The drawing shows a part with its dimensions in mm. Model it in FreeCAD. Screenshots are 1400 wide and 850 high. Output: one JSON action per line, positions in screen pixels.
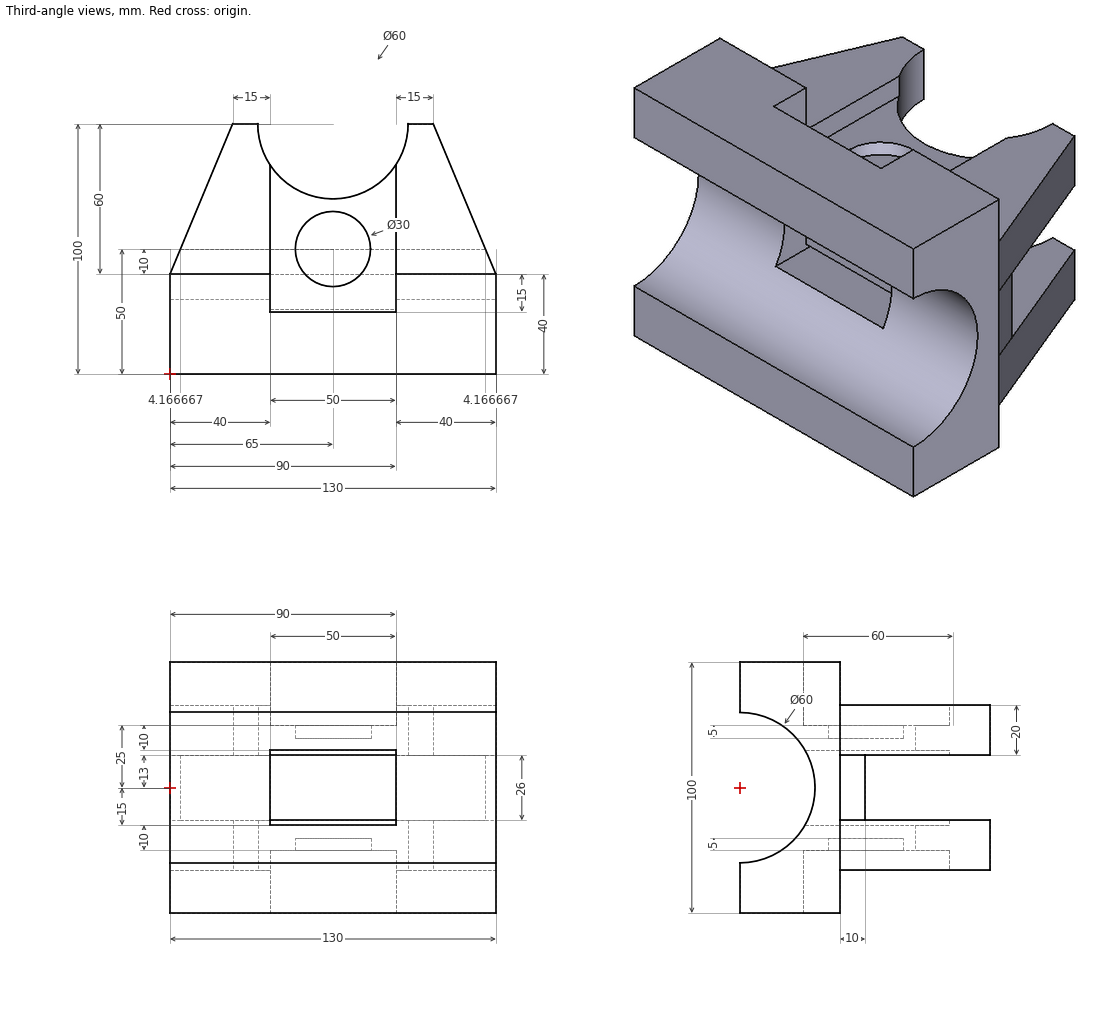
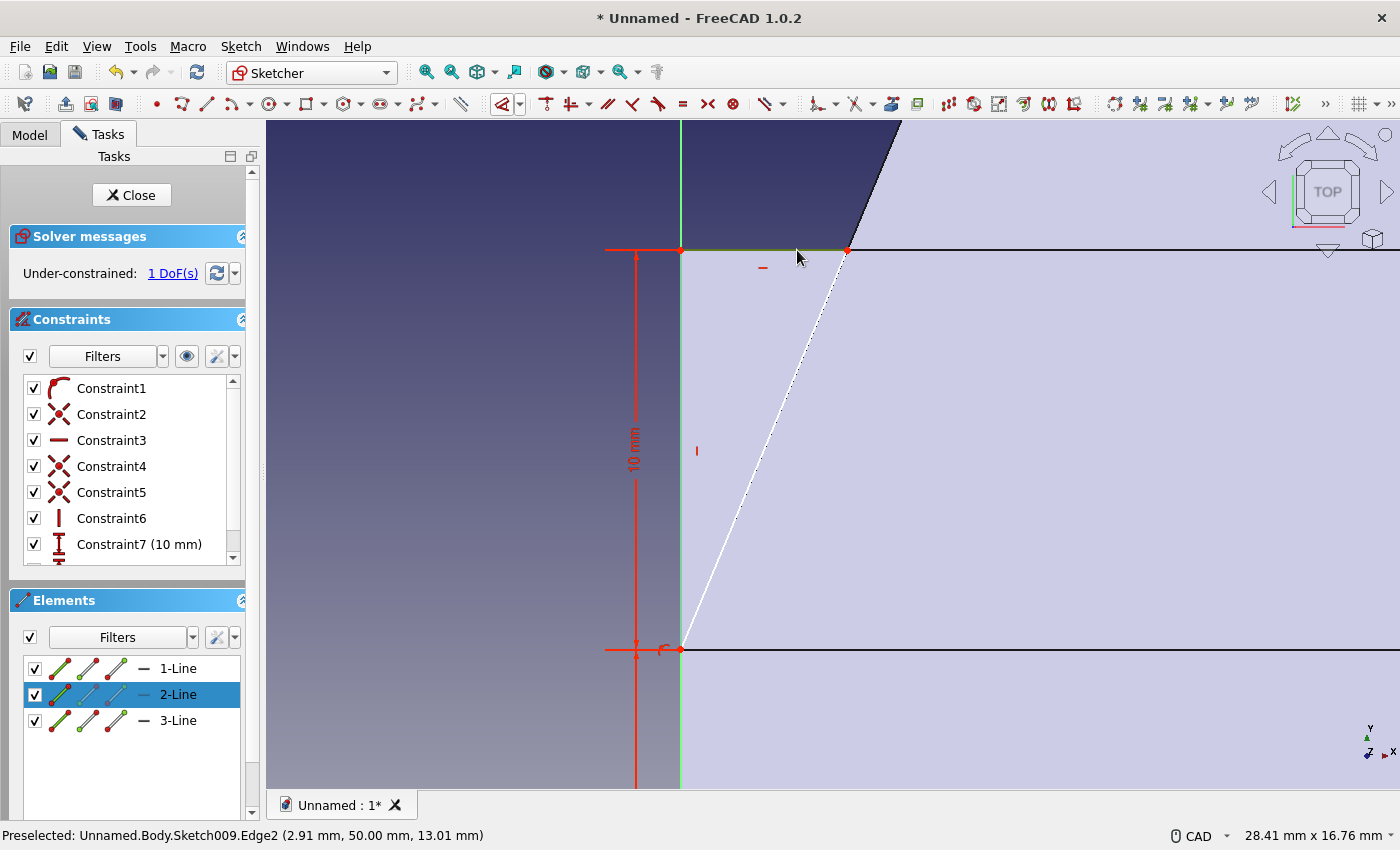
{"action": "left_click", "coordinate": [520, 104]}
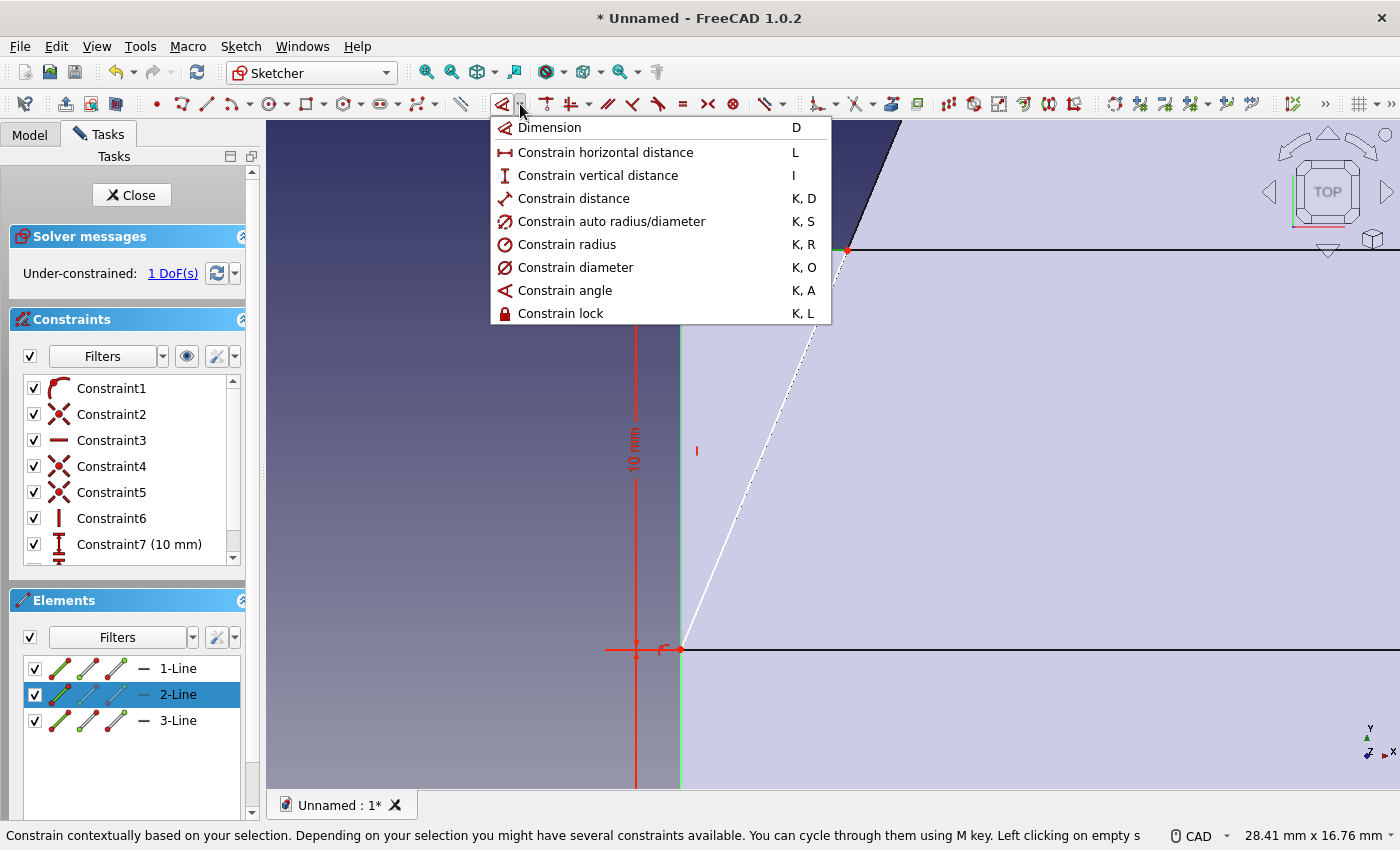
{"action": "left_click", "coordinate": [661, 152]}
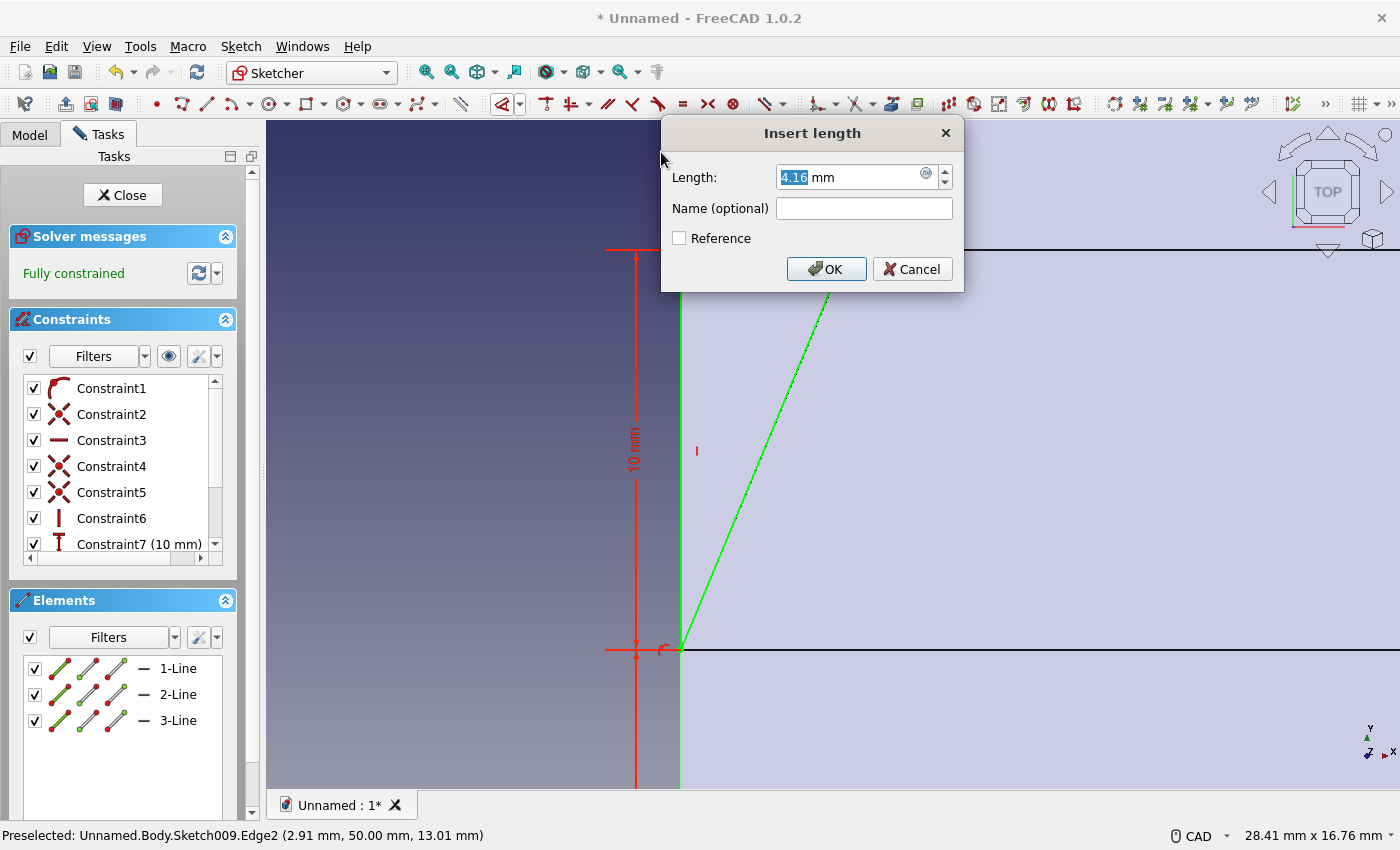
{"action": "type", "text": "4.166667"}
{"action": "key", "text": "Return"}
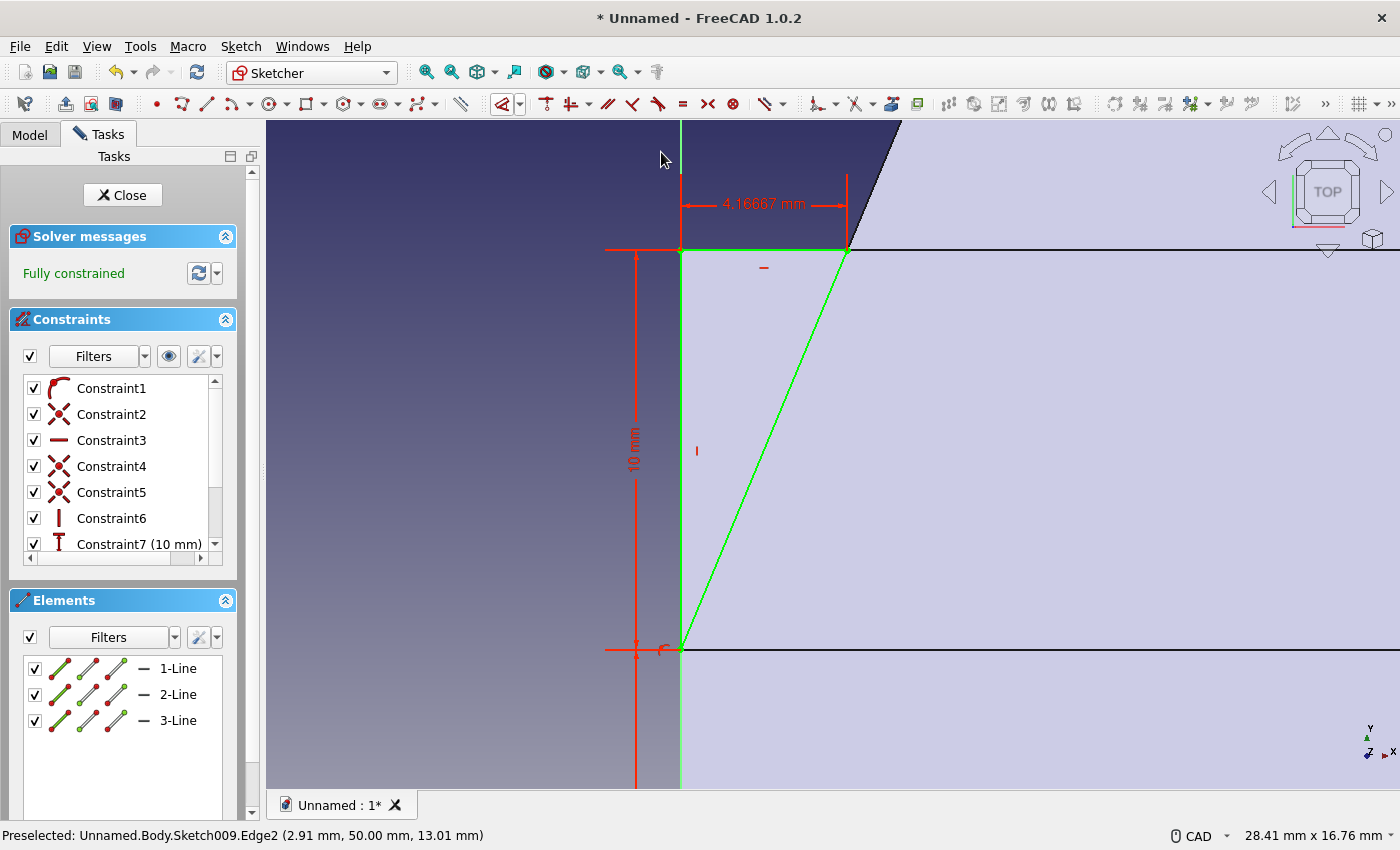
{"action": "left_click", "coordinate": [123, 195]}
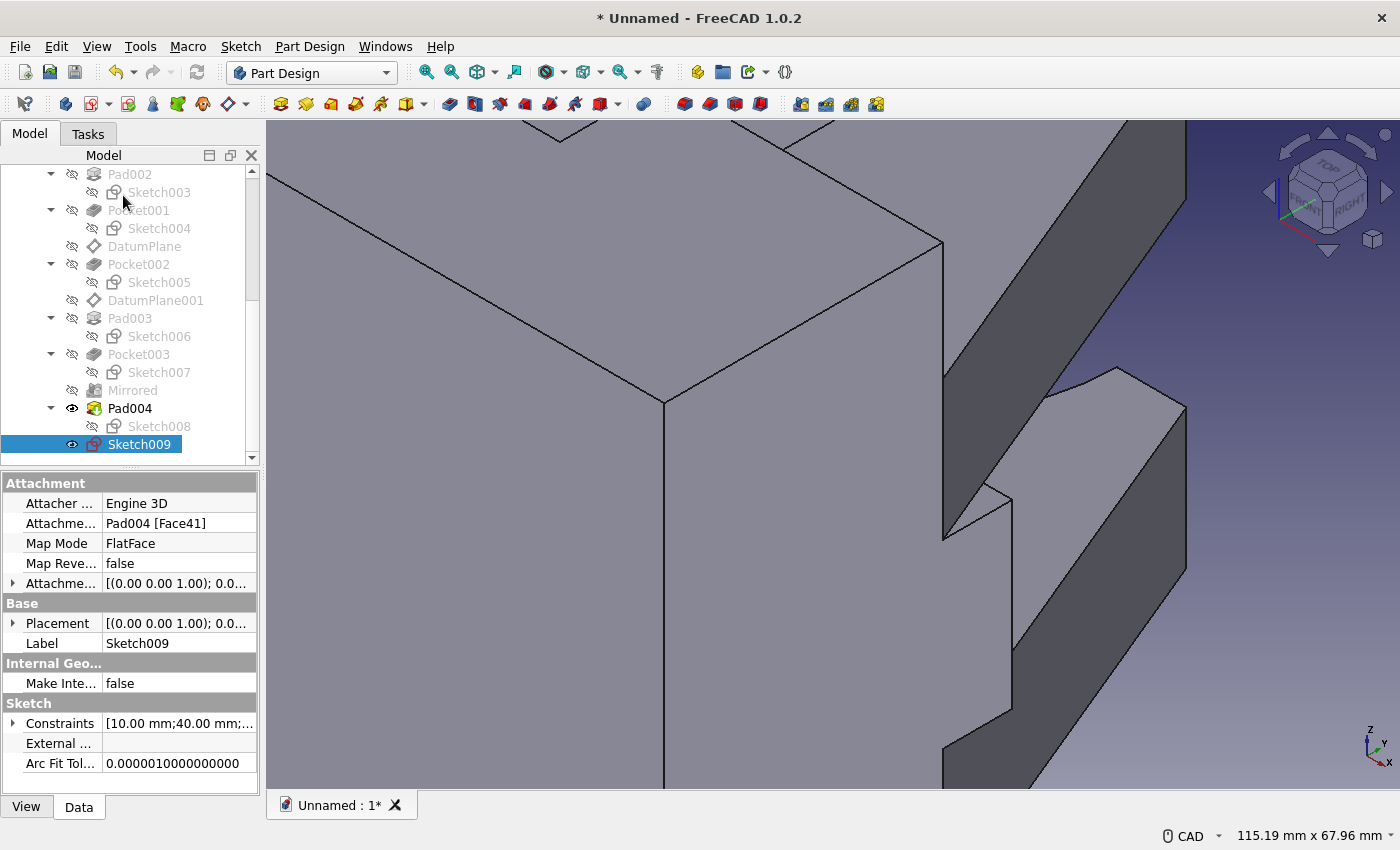
{"action": "left_click", "coordinate": [450, 104]}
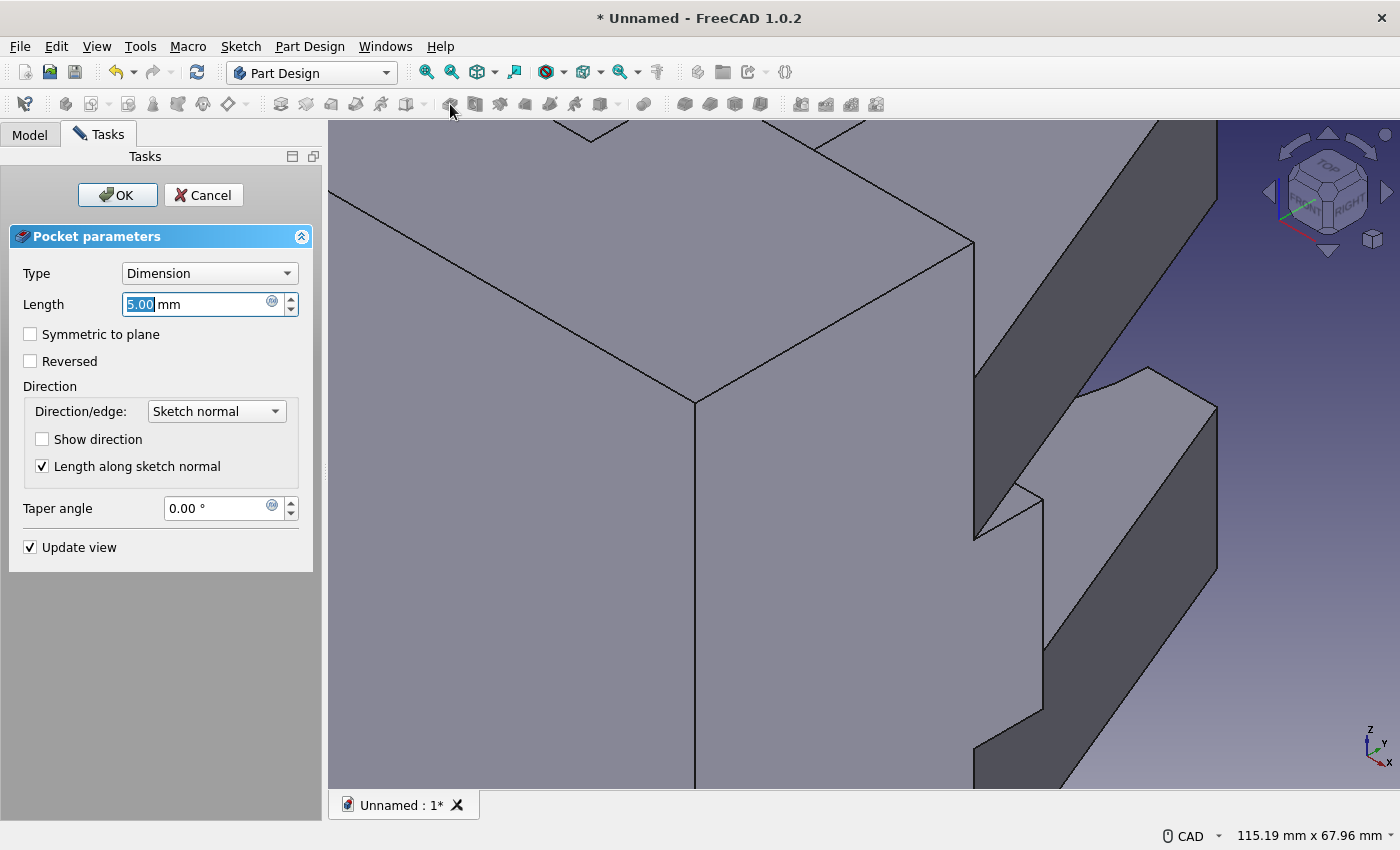
{"action": "left_click", "coordinate": [210, 274]}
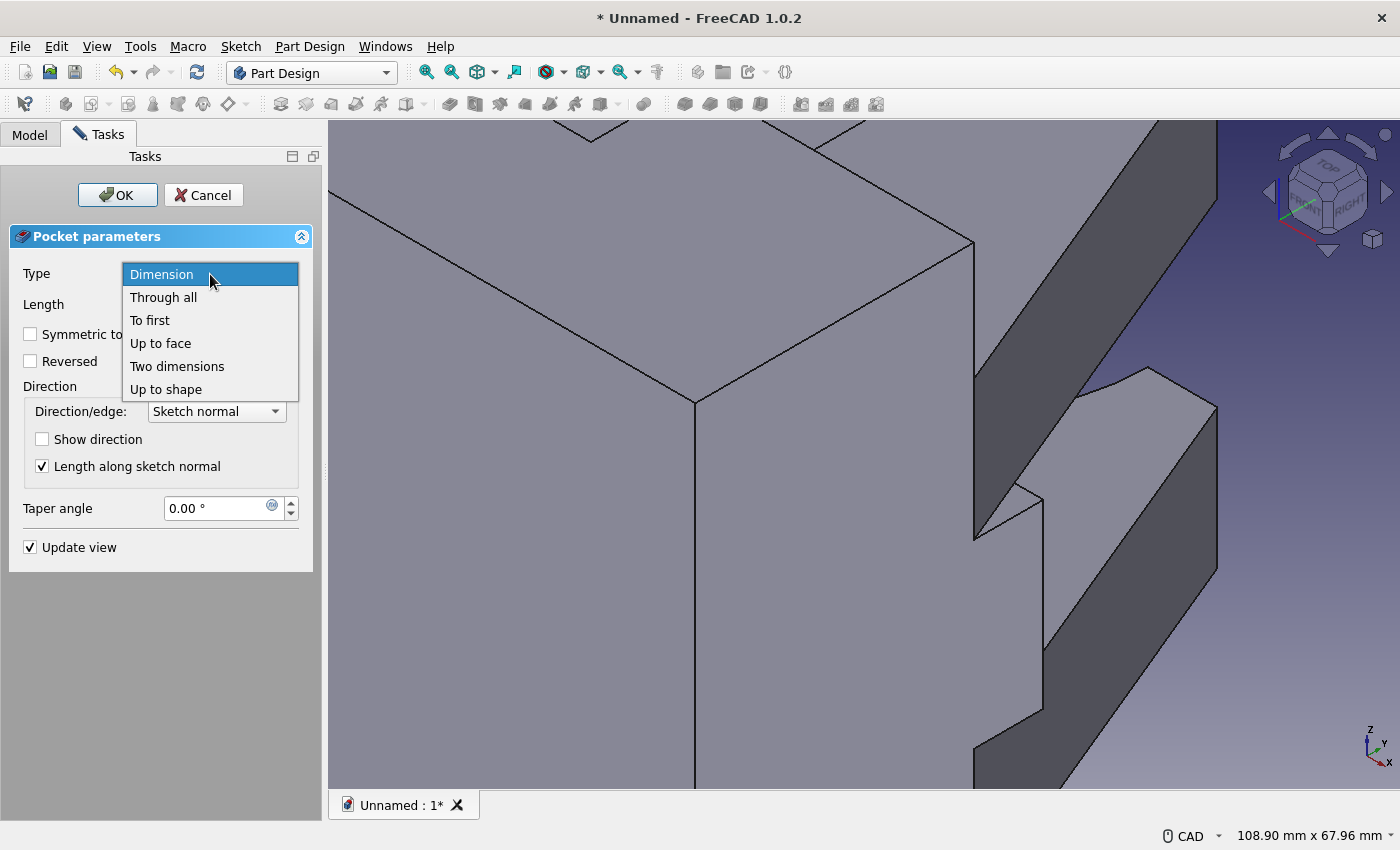
{"action": "left_click", "coordinate": [208, 298]}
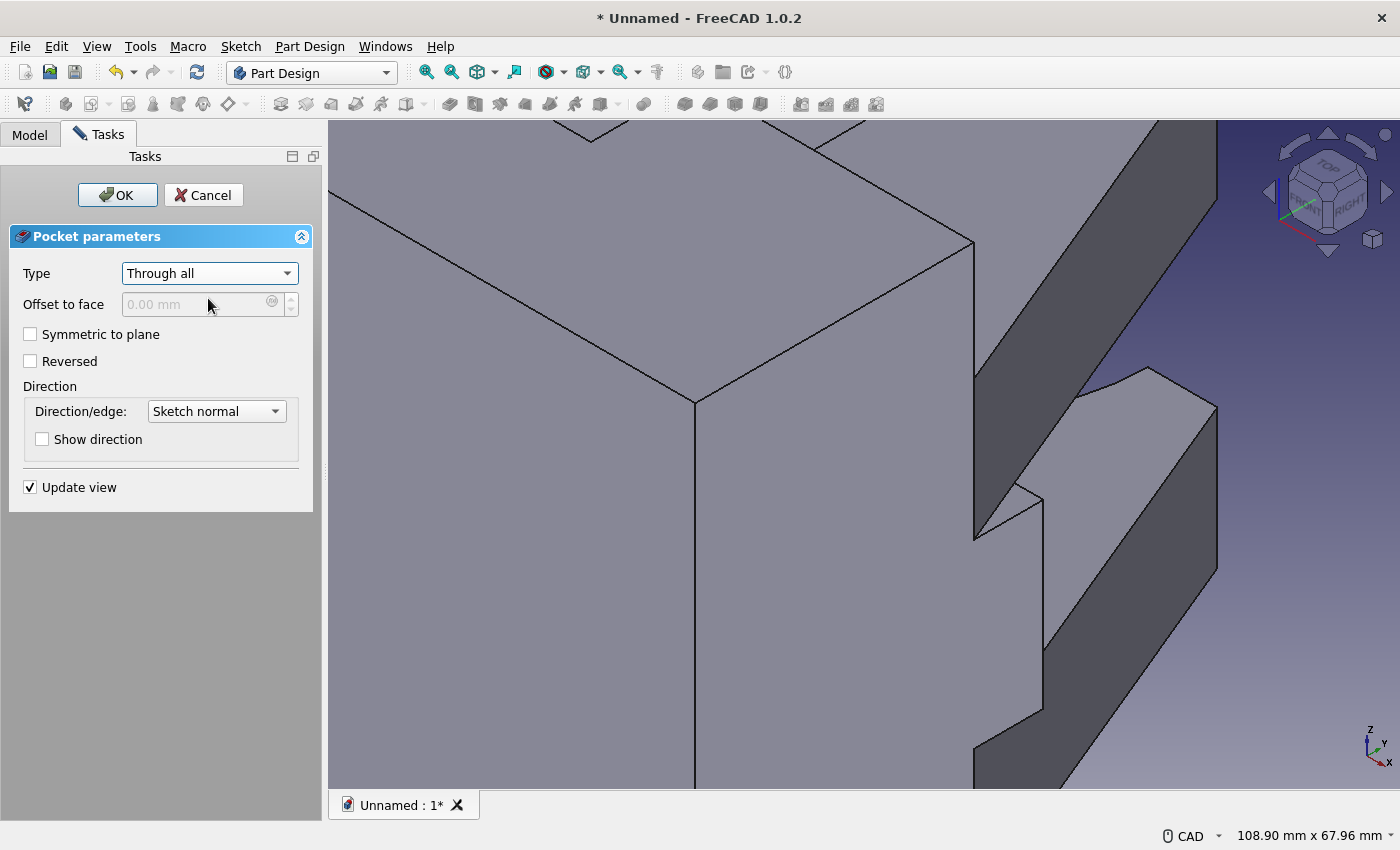
{"action": "left_click", "coordinate": [118, 195]}